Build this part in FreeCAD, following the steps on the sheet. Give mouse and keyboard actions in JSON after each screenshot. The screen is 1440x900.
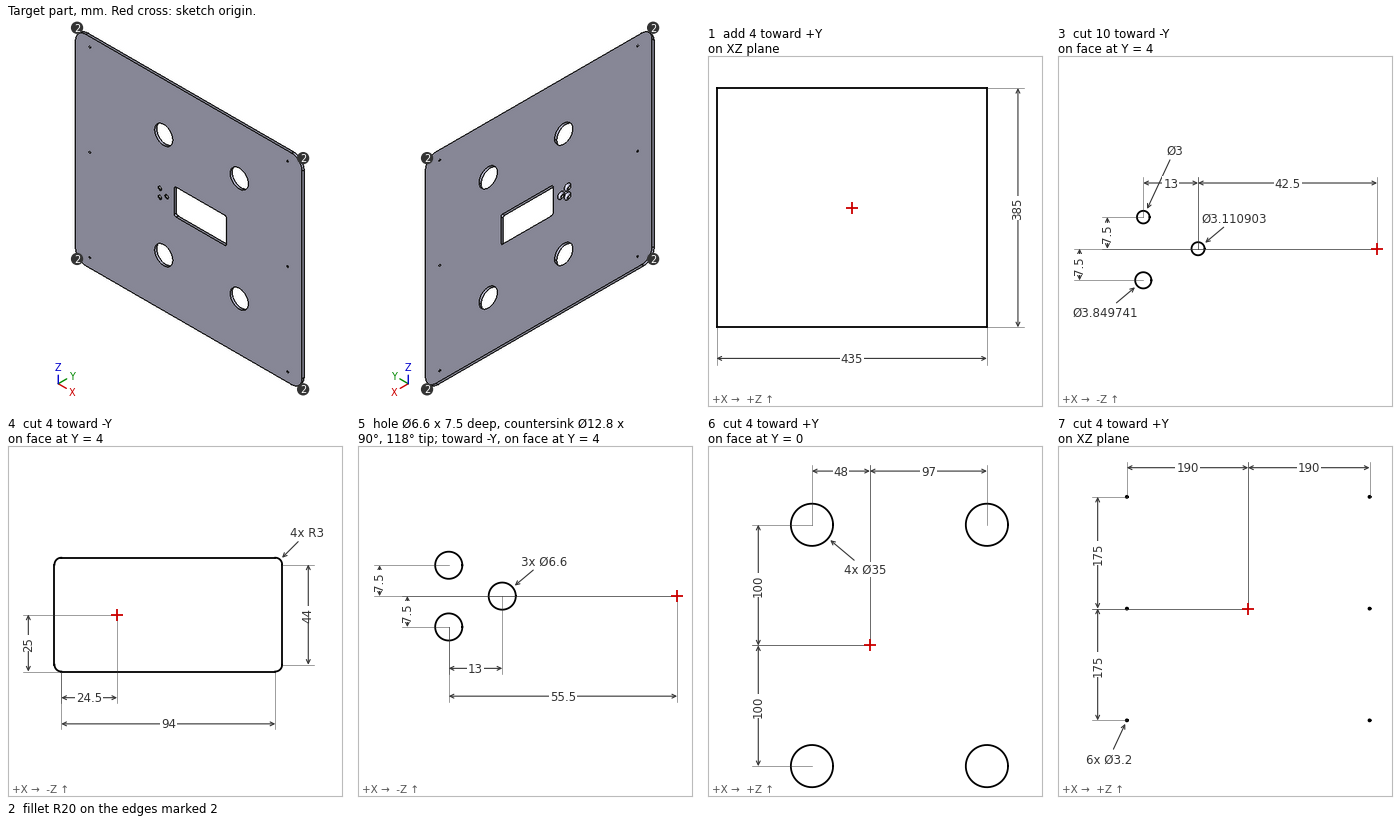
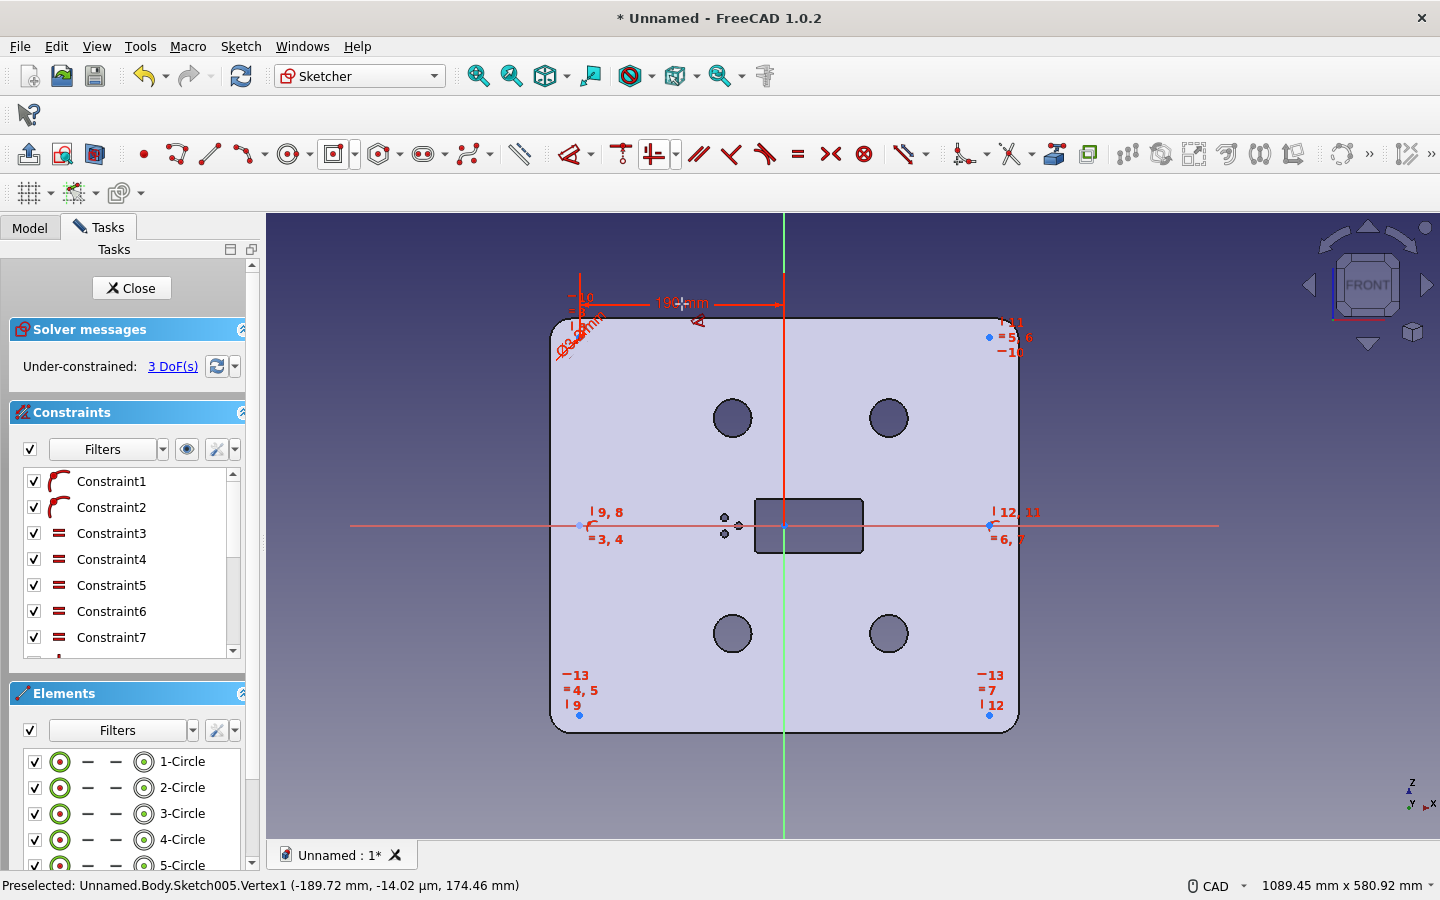
{"action": "left_click", "coordinate": [580, 338]}
{"action": "left_click", "coordinate": [546, 432]}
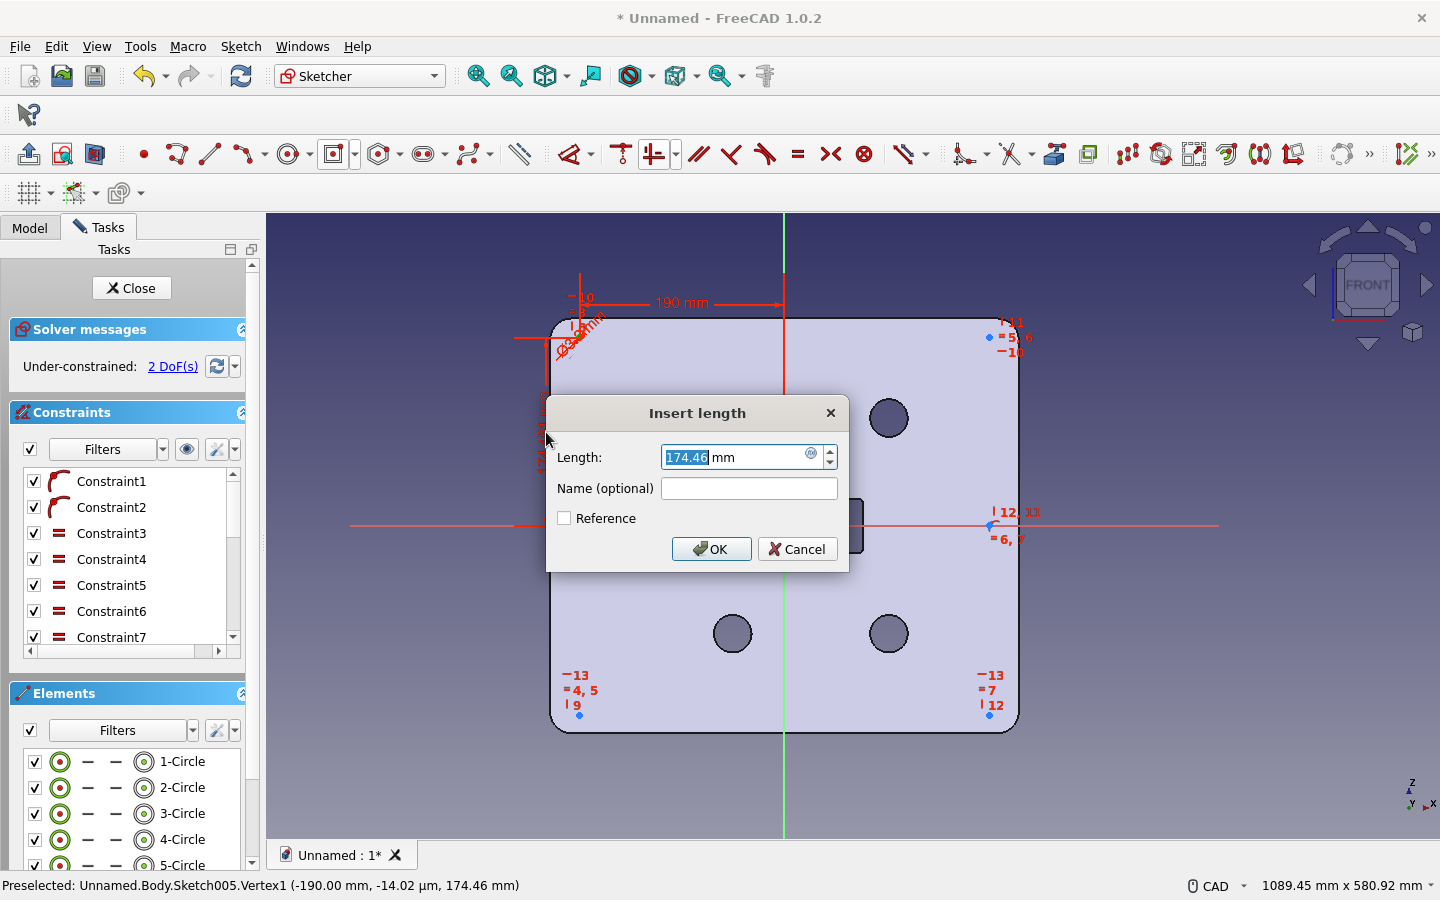
{"action": "type", "text": "175"}
{"action": "key", "text": "Return"}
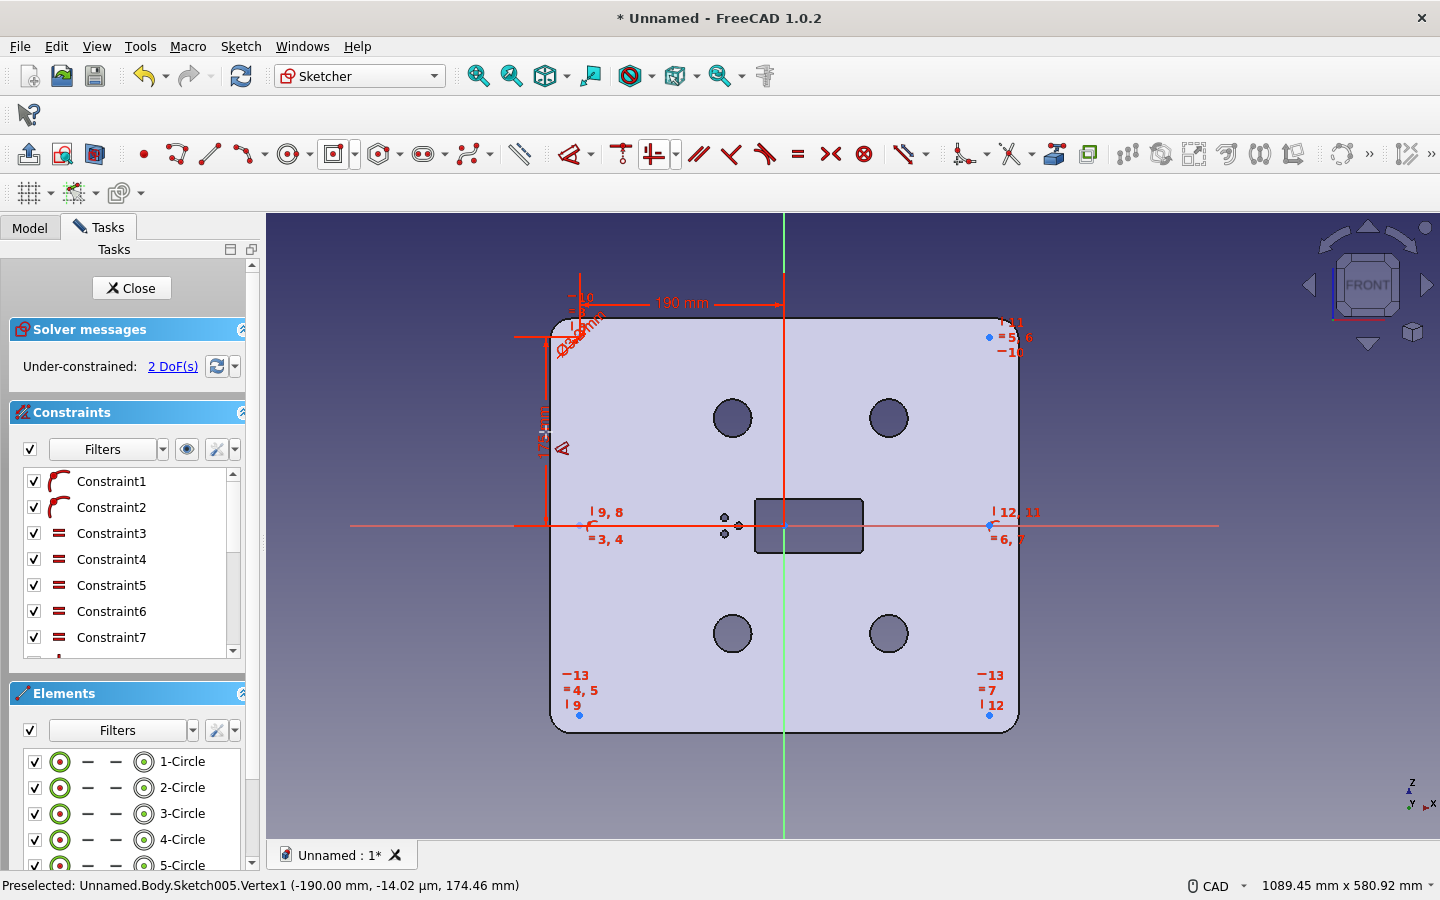
{"action": "left_click", "coordinate": [580, 716]}
{"action": "left_click", "coordinate": [546, 621]}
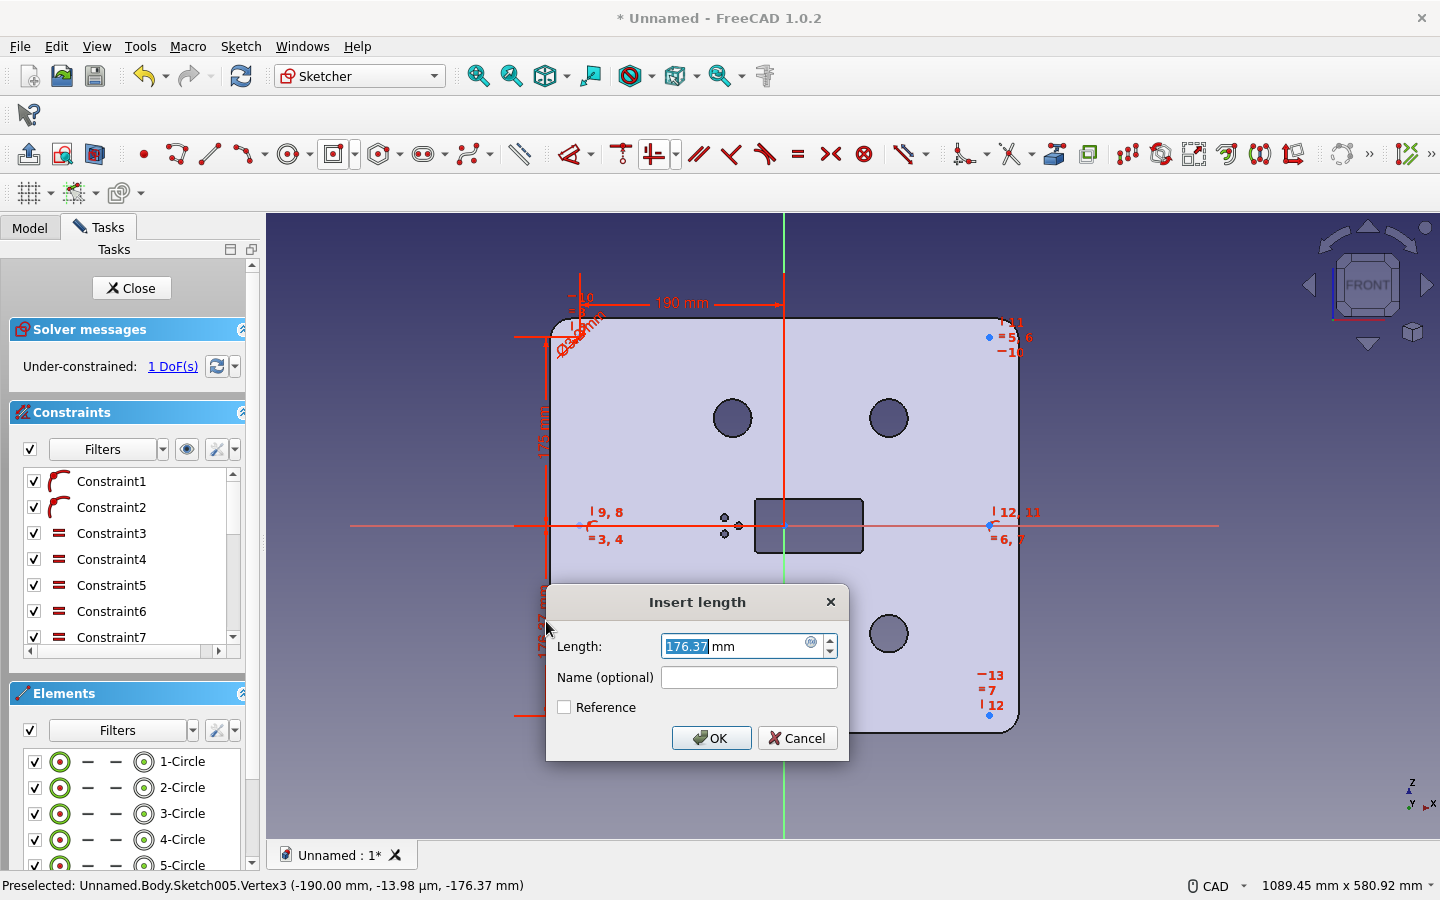
{"action": "type", "text": "175"}
{"action": "key", "text": "Return"}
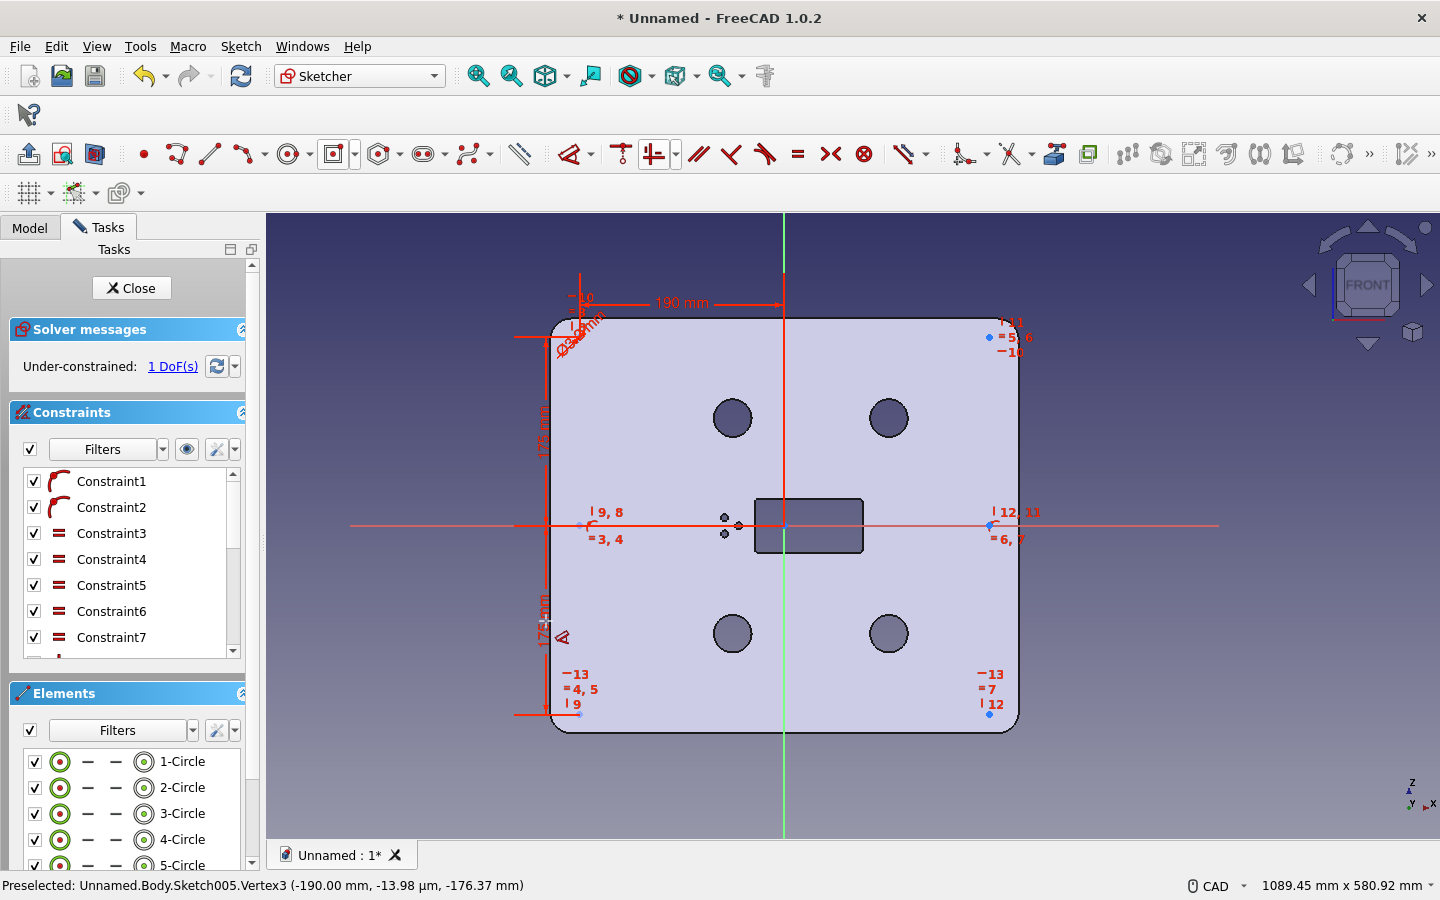
{"action": "left_click", "coordinate": [989, 337]}
{"action": "left_click", "coordinate": [887, 303]}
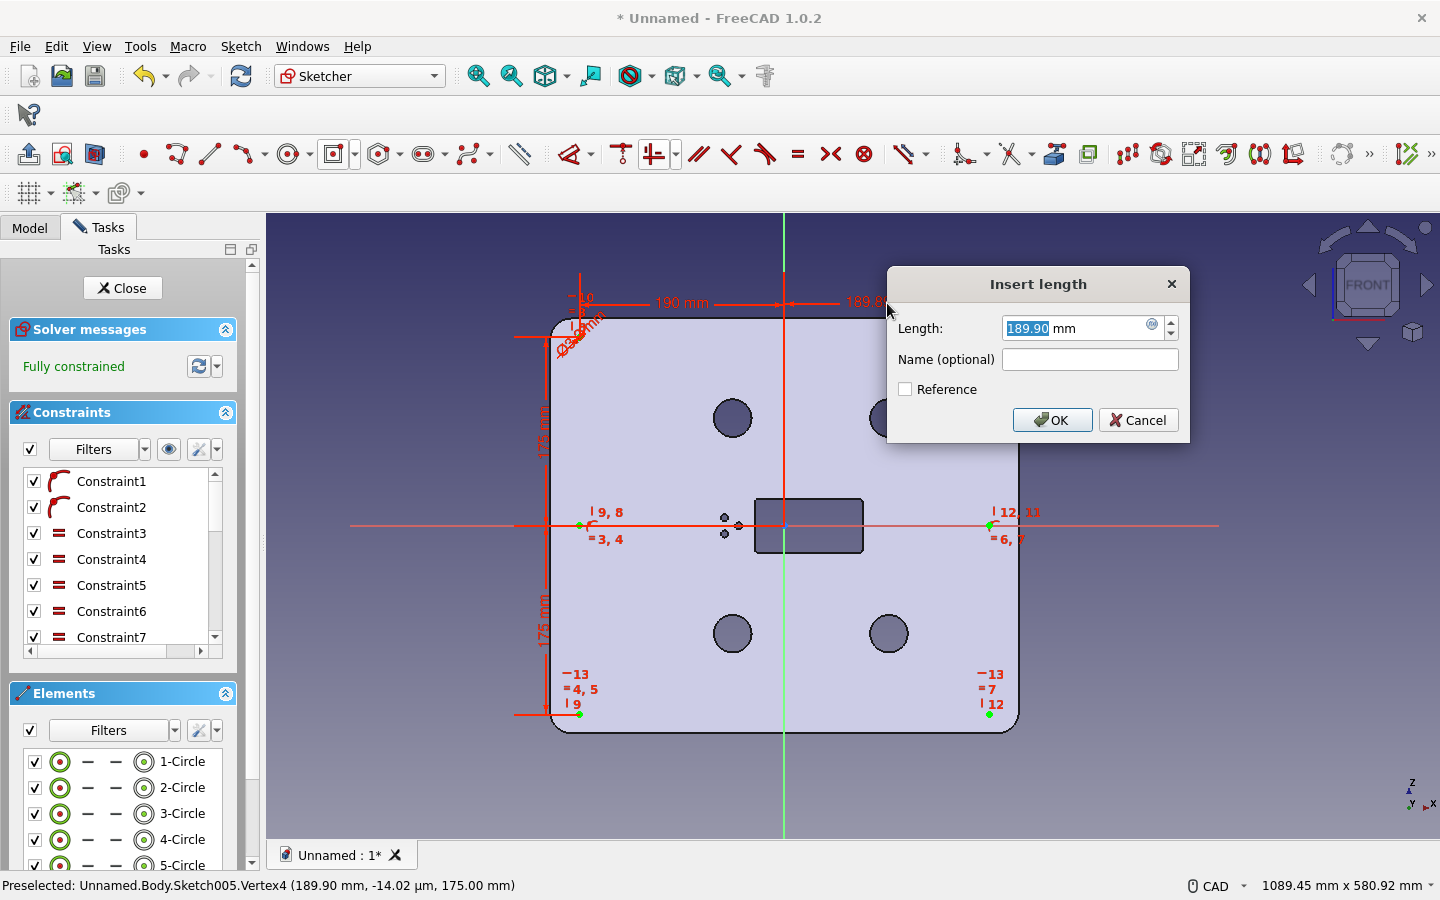
{"action": "type", "text": "190"}
{"action": "key", "text": "Return"}
{"action": "key", "text": "Escape"}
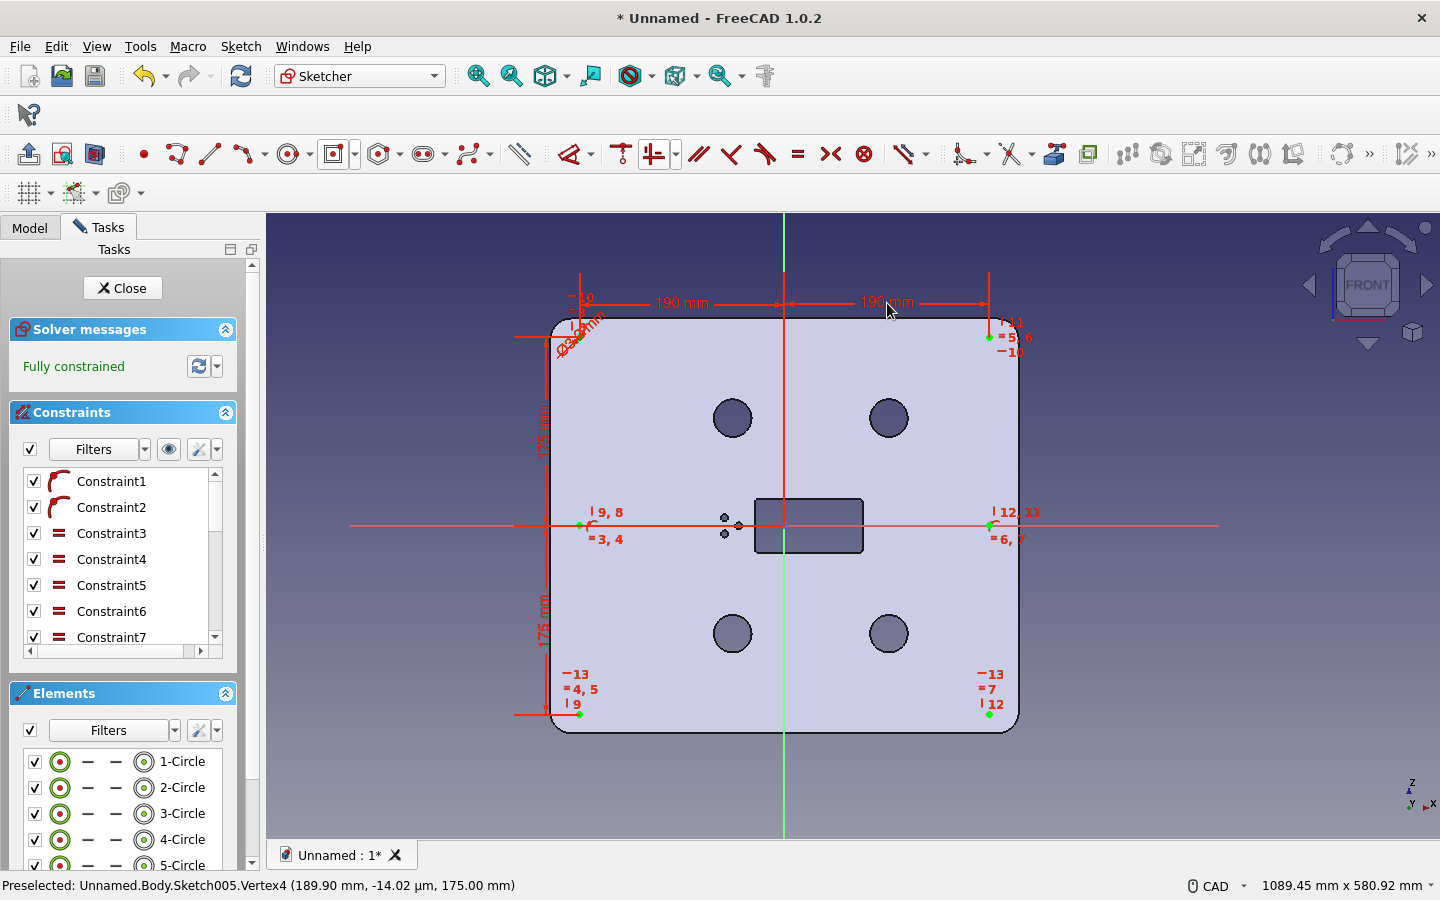
{"action": "left_click", "coordinate": [123, 288]}